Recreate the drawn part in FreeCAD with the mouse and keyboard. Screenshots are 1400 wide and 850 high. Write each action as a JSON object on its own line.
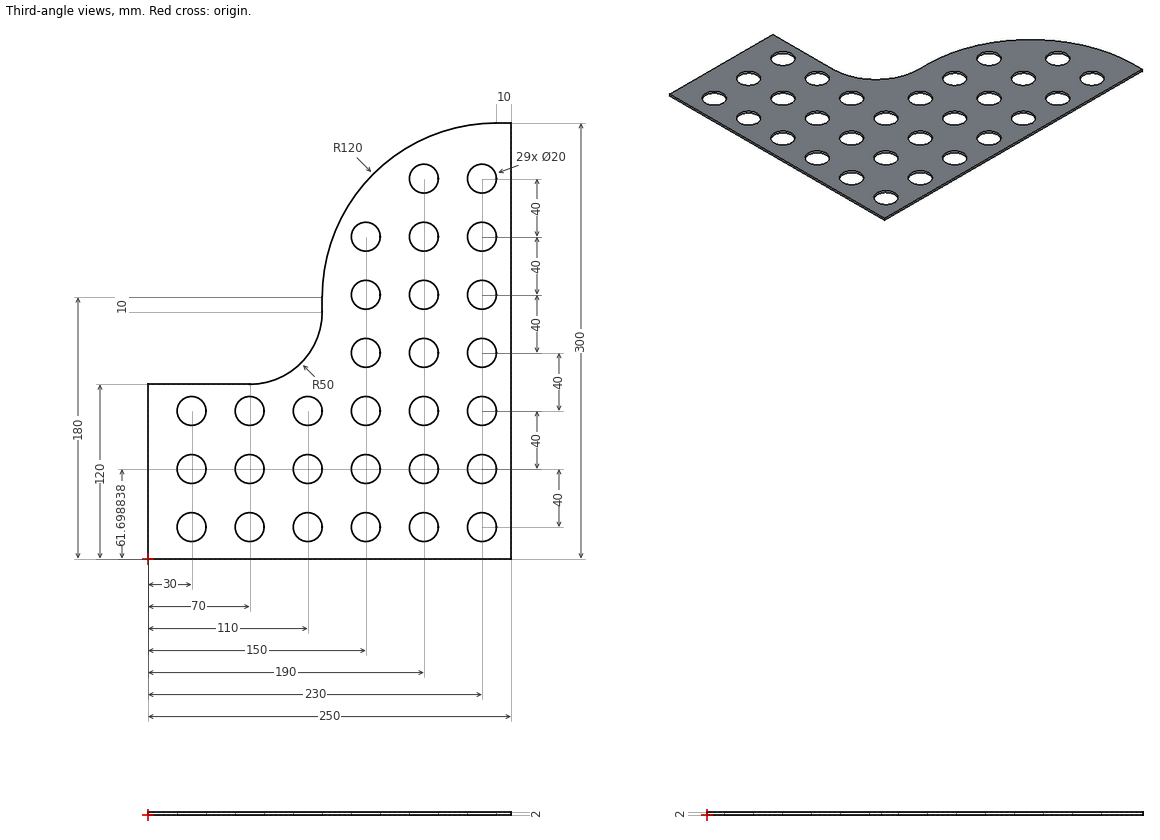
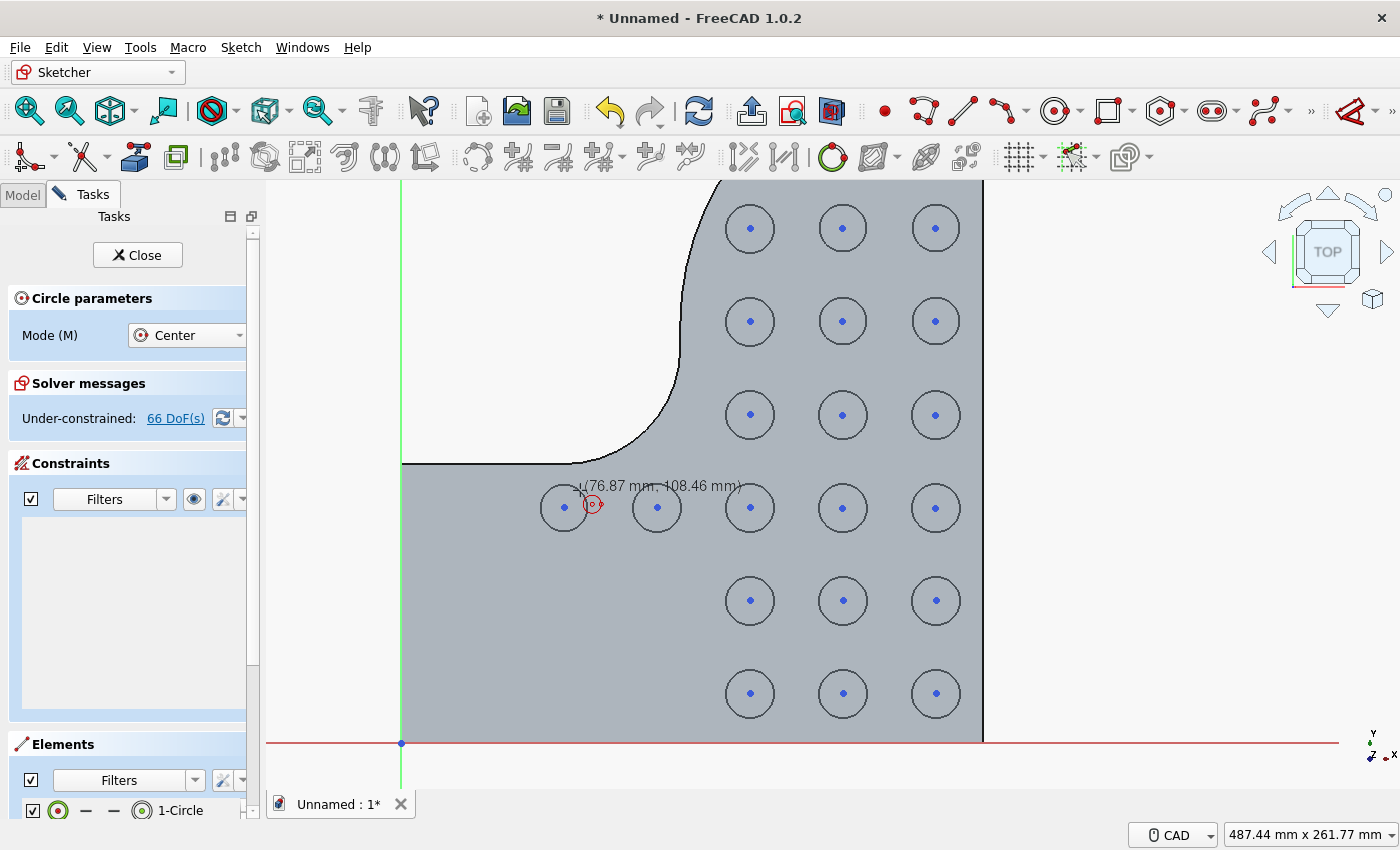
{"action": "left_click", "coordinate": [471, 507]}
{"action": "left_click", "coordinate": [487, 490]}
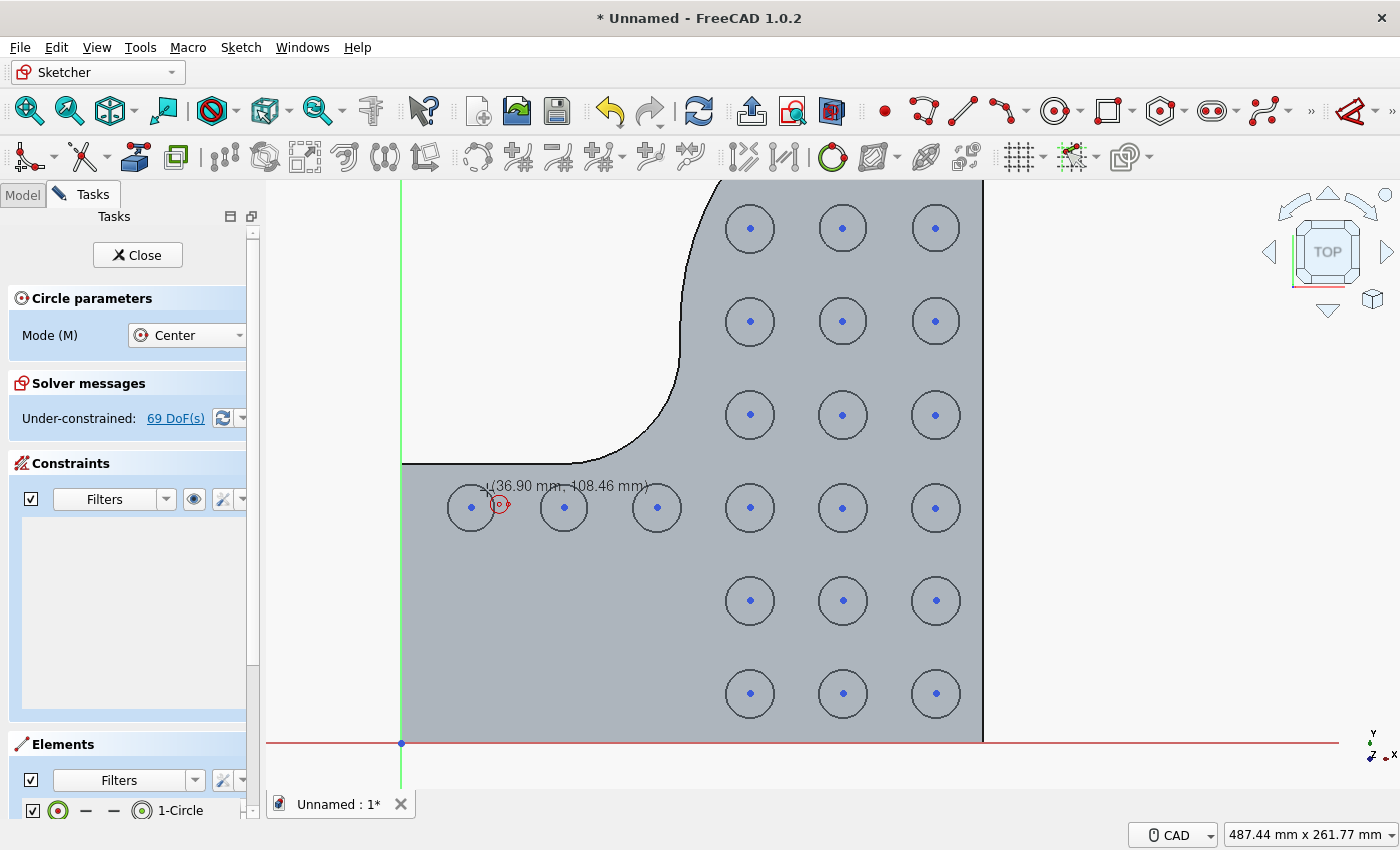
{"action": "left_click", "coordinate": [657, 600]}
{"action": "left_click", "coordinate": [674, 583]}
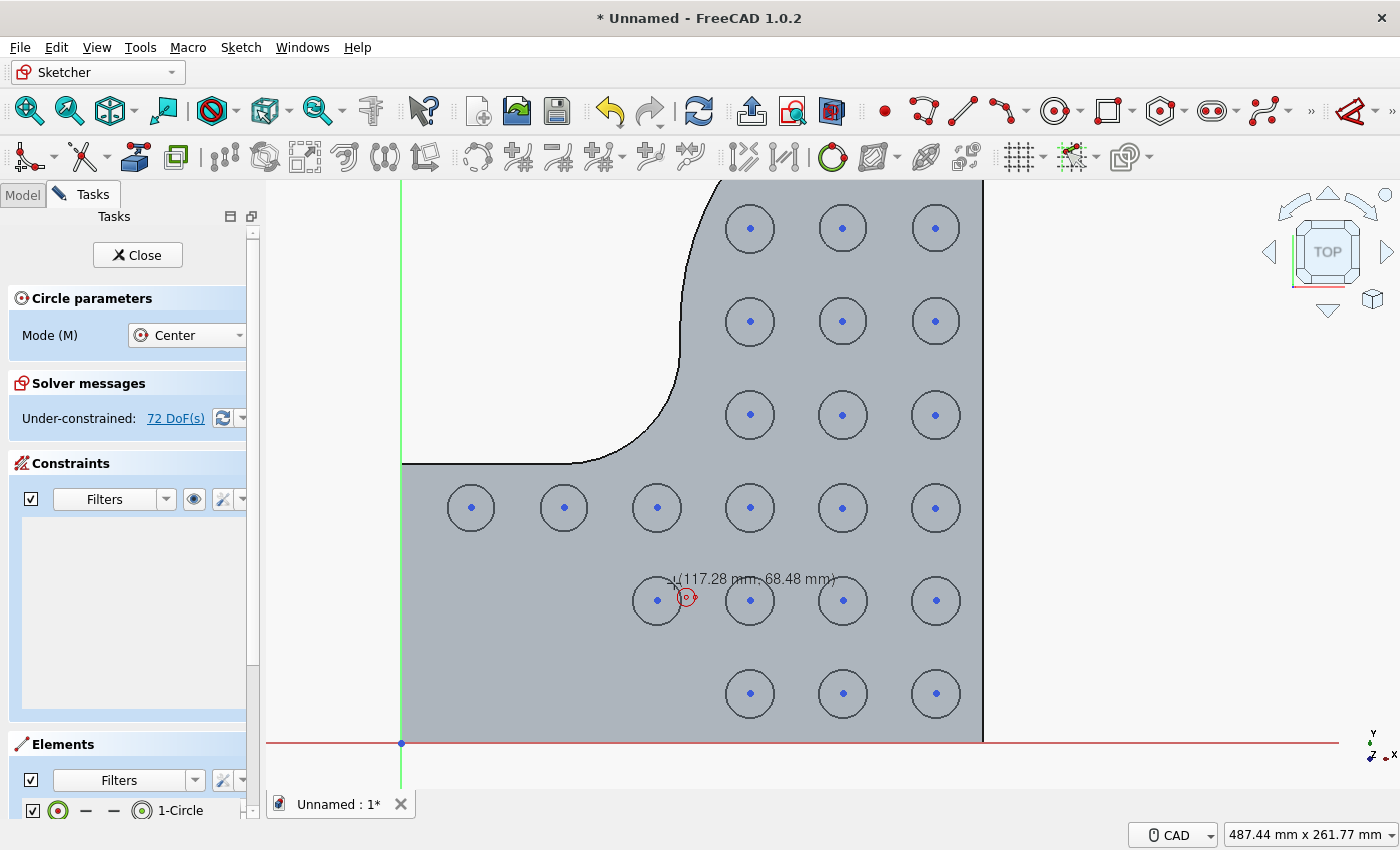
{"action": "left_click", "coordinate": [564, 600]}
{"action": "left_click", "coordinate": [580, 583]}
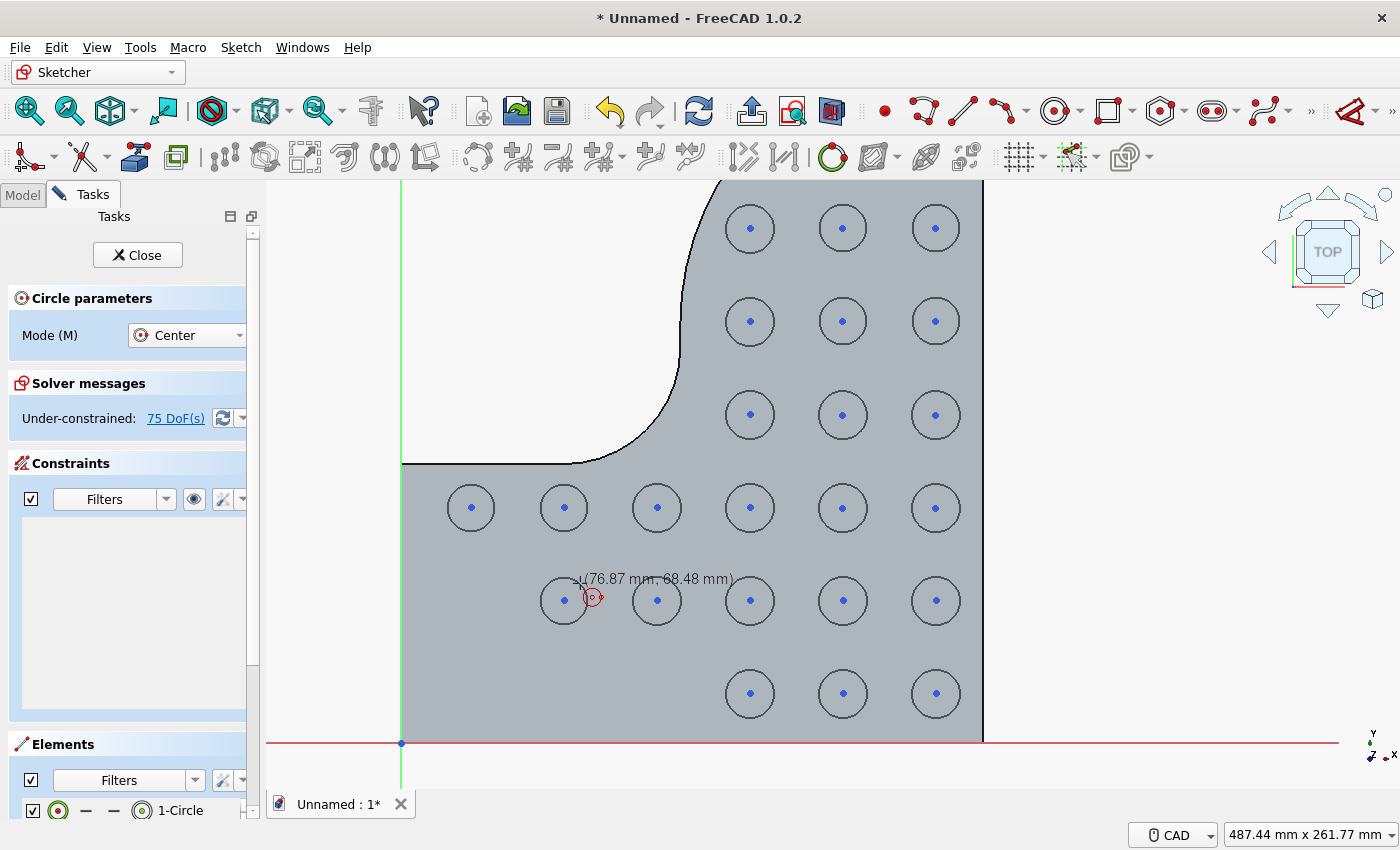
{"action": "left_click", "coordinate": [471, 600]}
{"action": "left_click", "coordinate": [487, 583]}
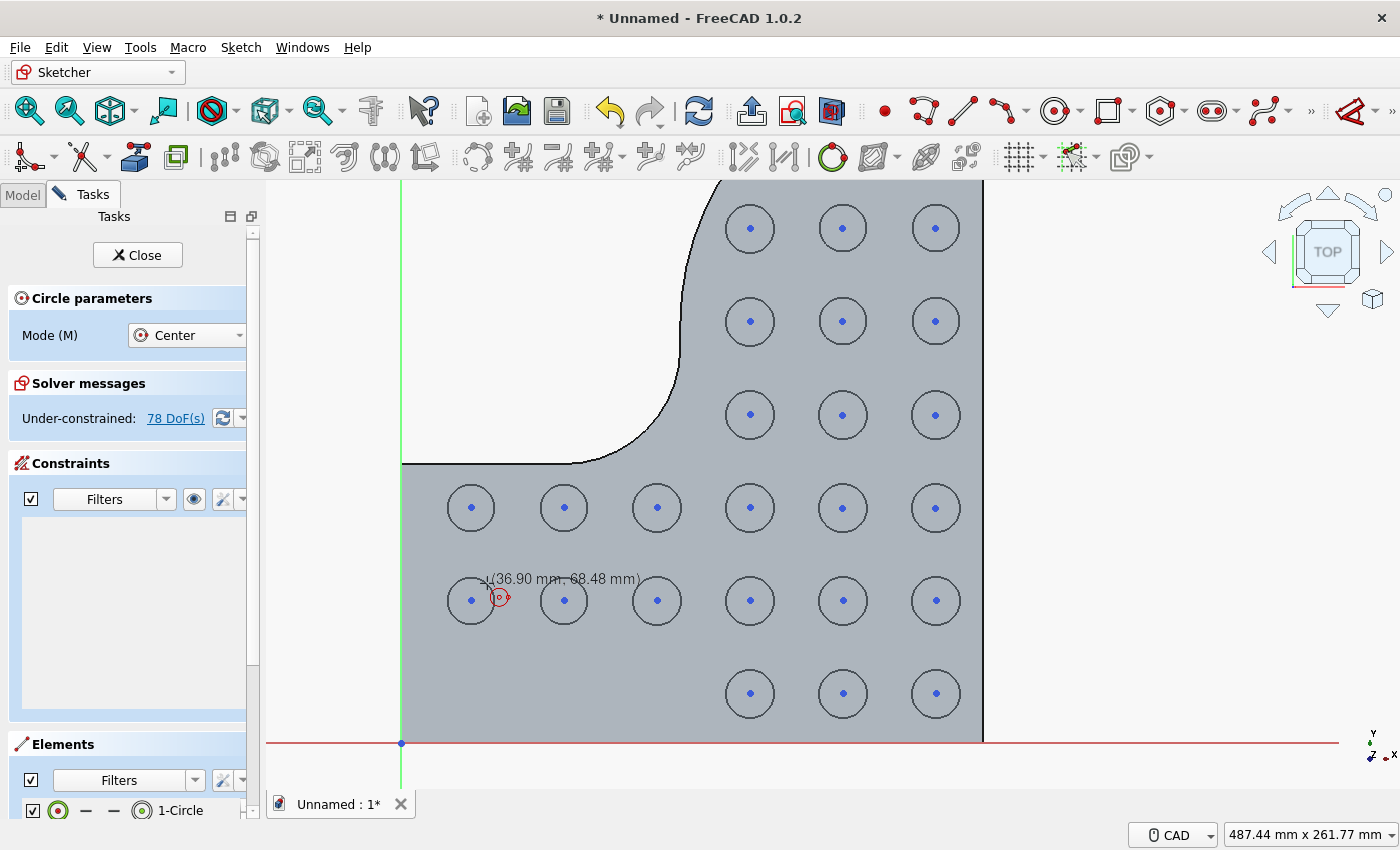
{"action": "left_click", "coordinate": [657, 693]}
{"action": "left_click", "coordinate": [674, 676]}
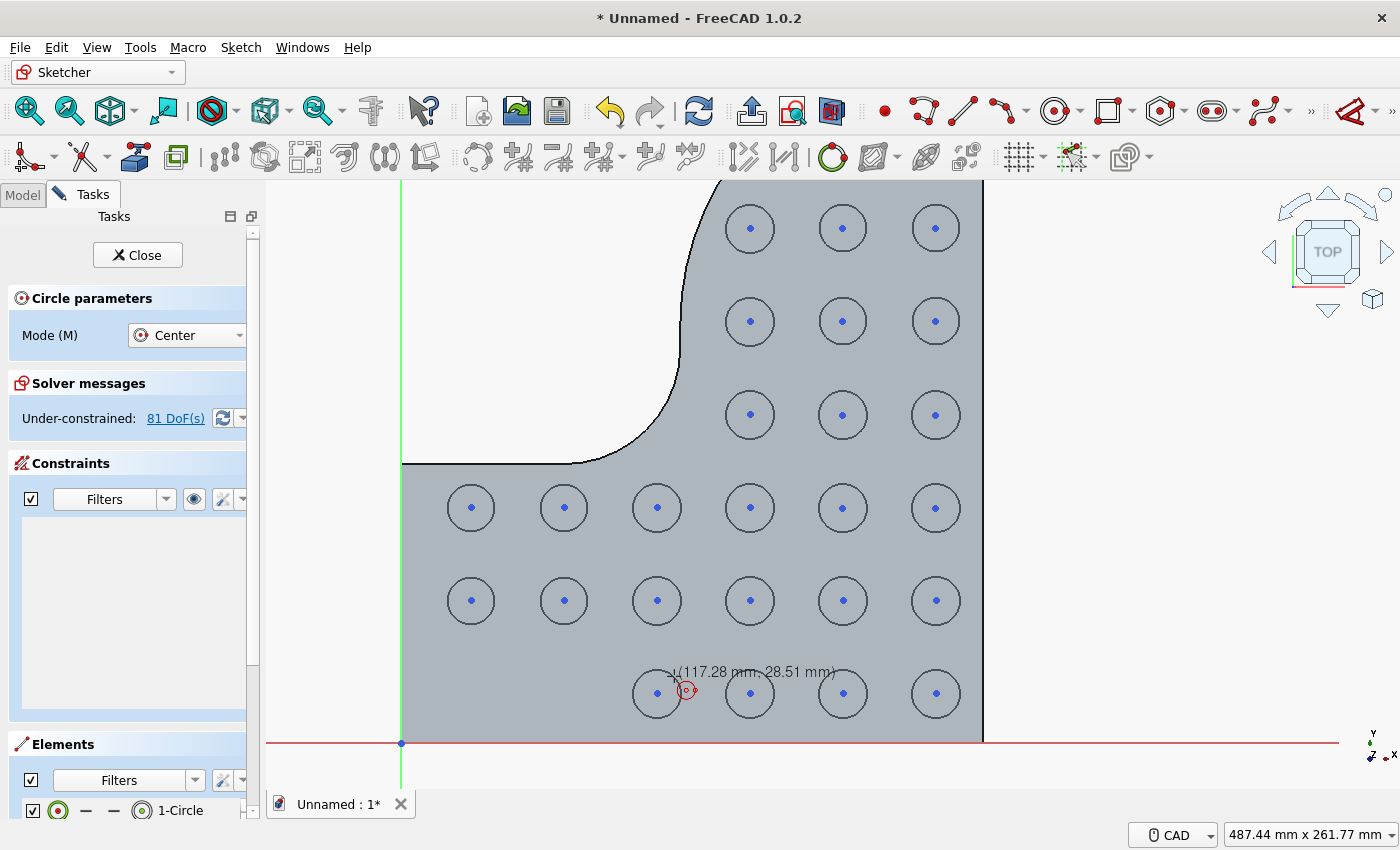
{"action": "left_click", "coordinate": [564, 693]}
{"action": "left_click", "coordinate": [580, 676]}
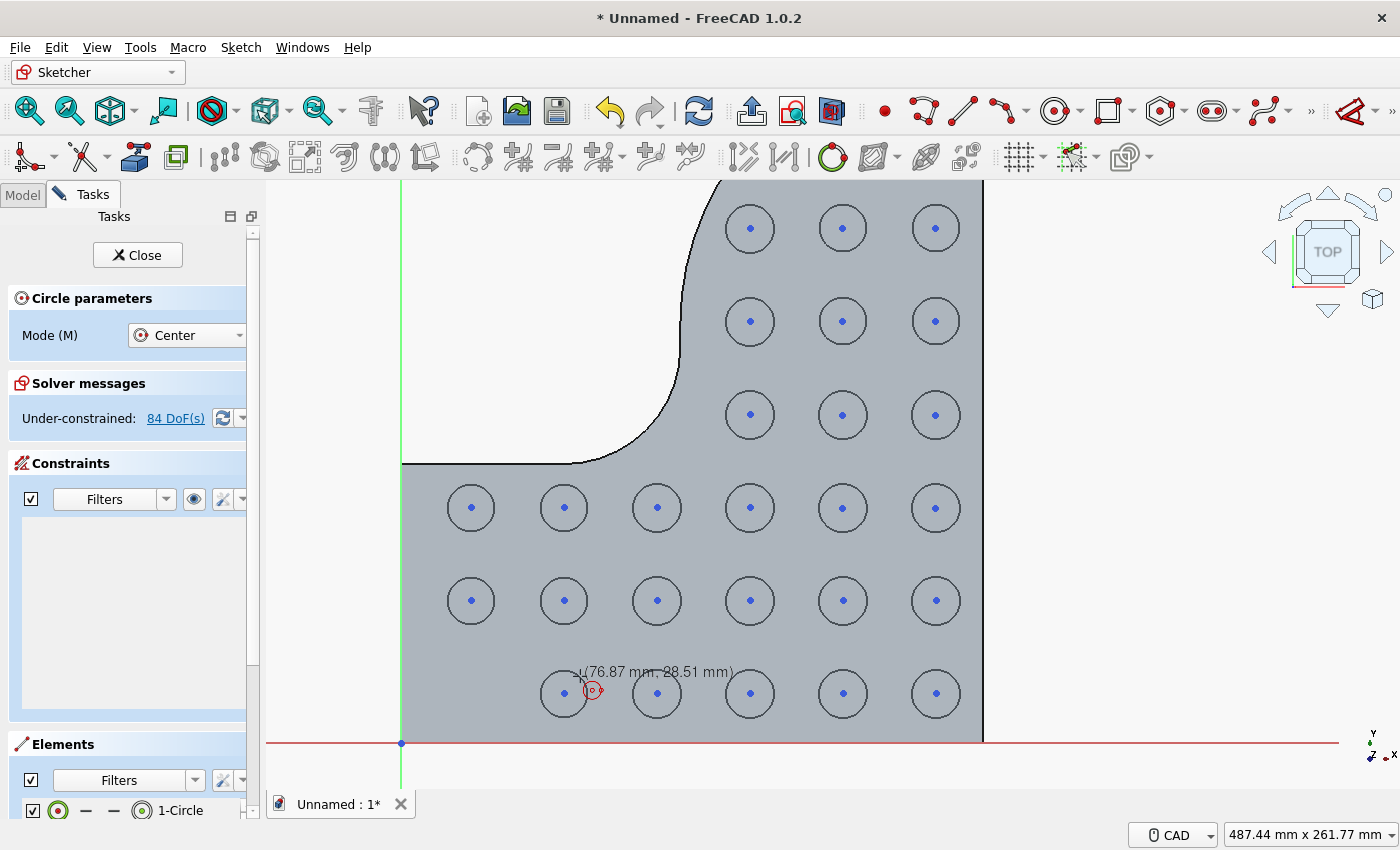
{"action": "left_click", "coordinate": [471, 693]}
{"action": "left_click", "coordinate": [487, 676]}
{"action": "key", "text": "Escape"}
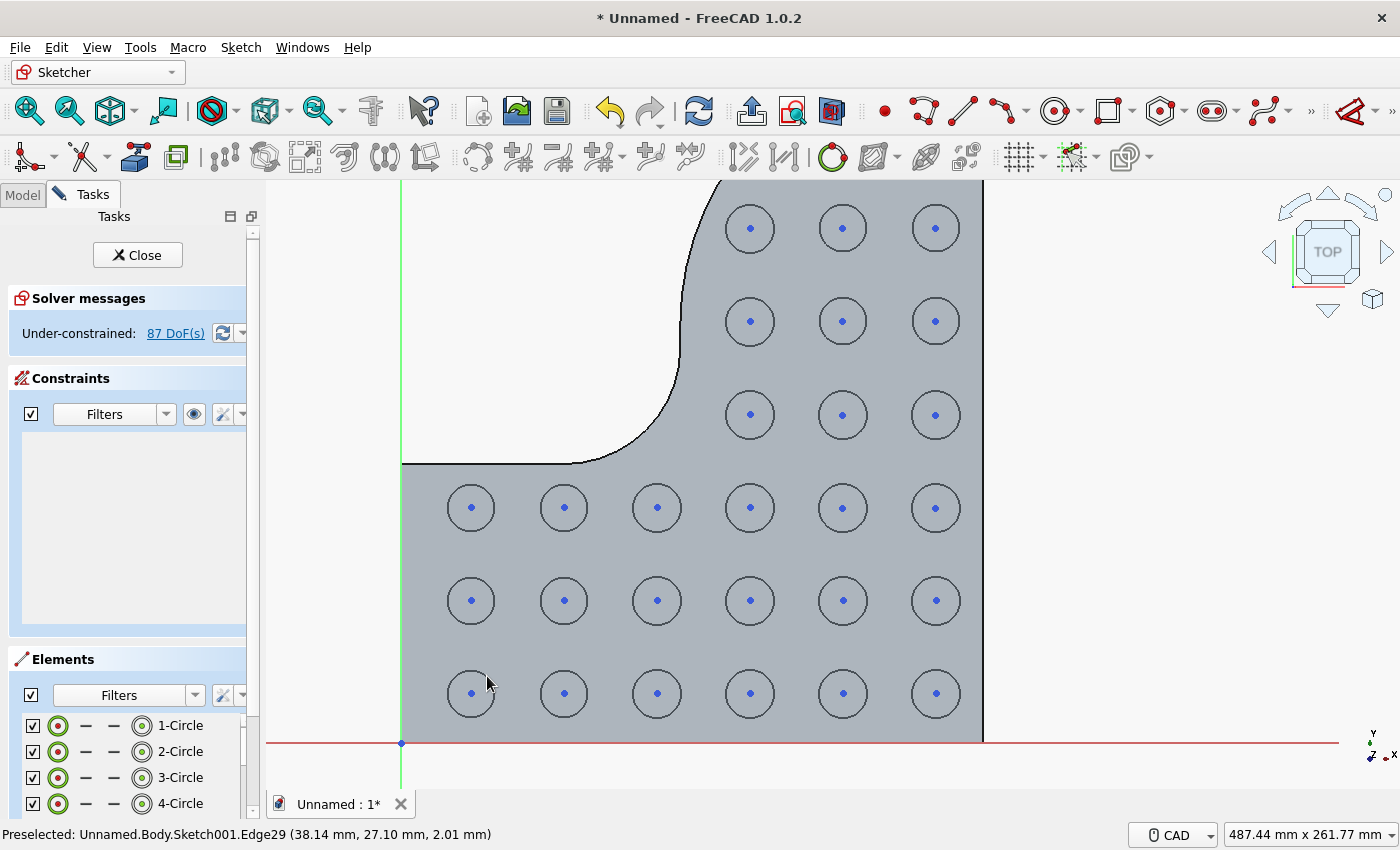
{"action": "scroll", "coordinate": [936, 601], "scroll_direction": "down", "scroll_amount": 2}